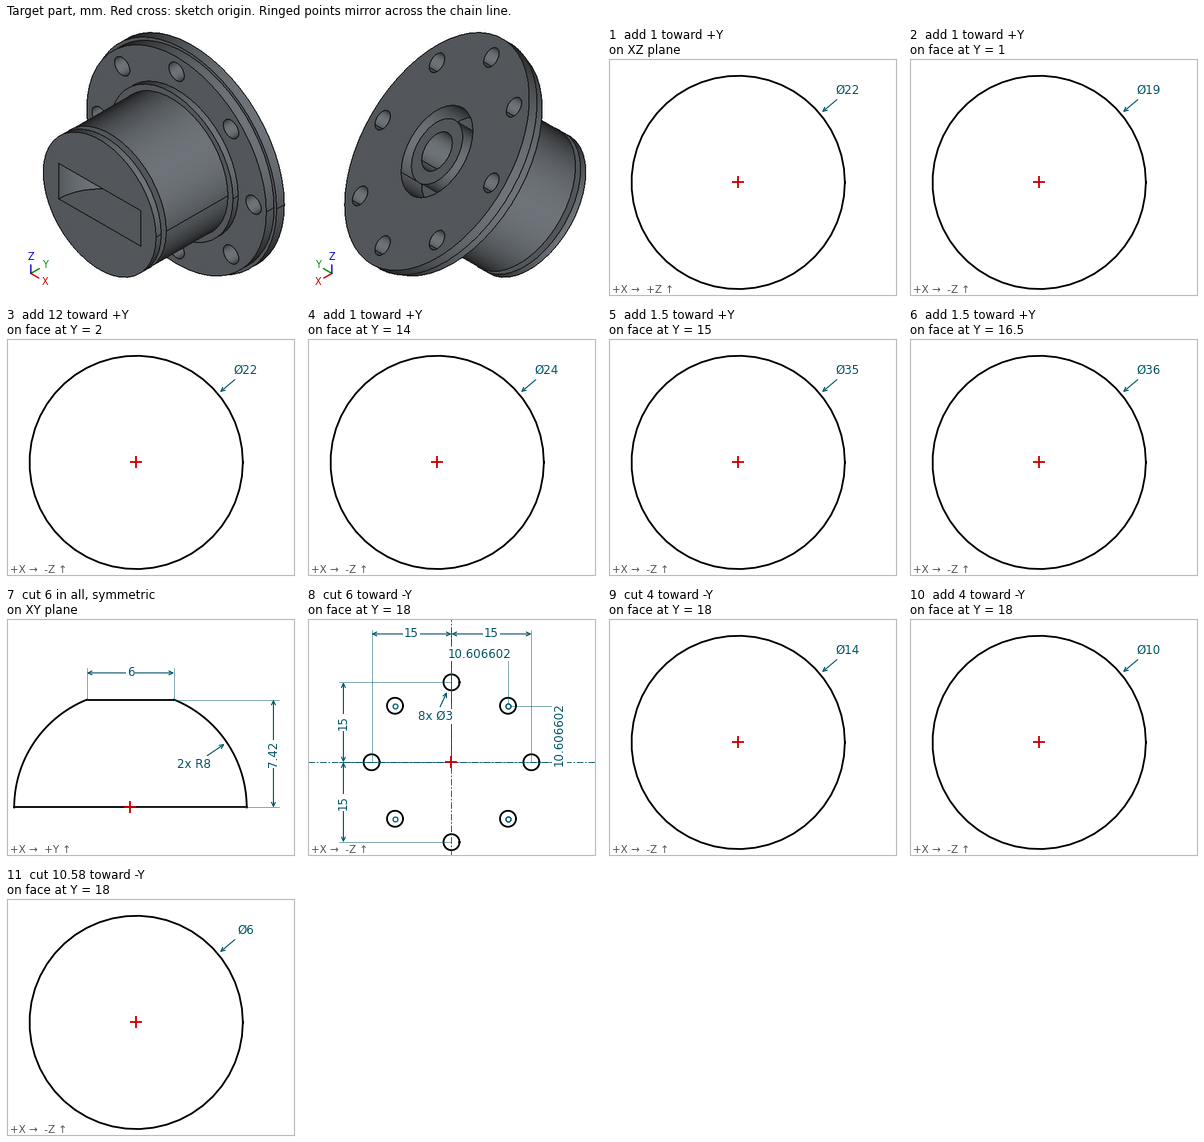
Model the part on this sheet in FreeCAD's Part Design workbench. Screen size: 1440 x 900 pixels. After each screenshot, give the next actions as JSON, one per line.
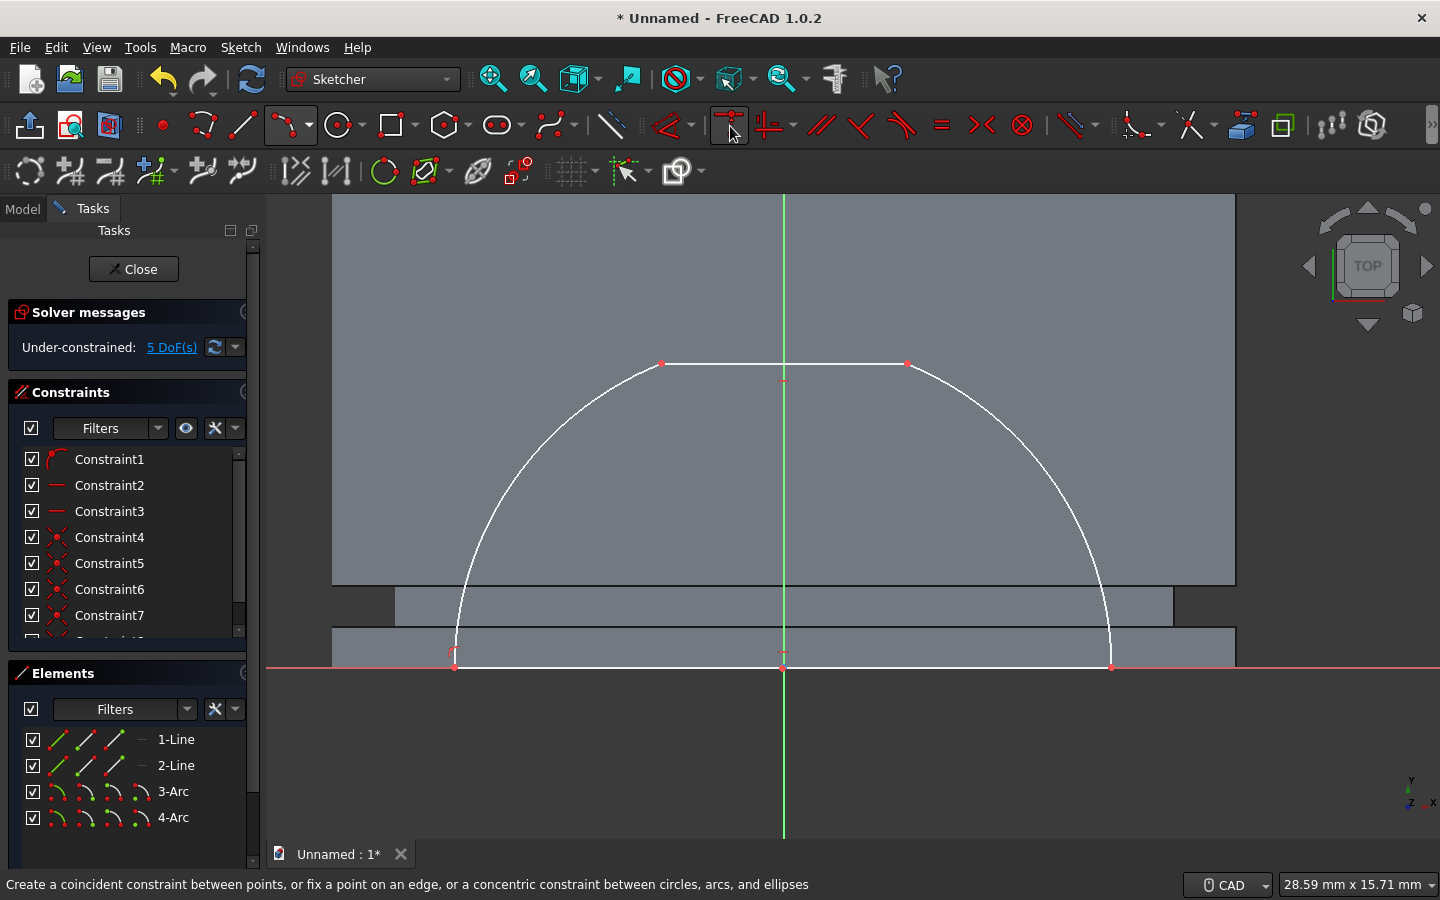
{"action": "left_click", "coordinate": [1091, 554]}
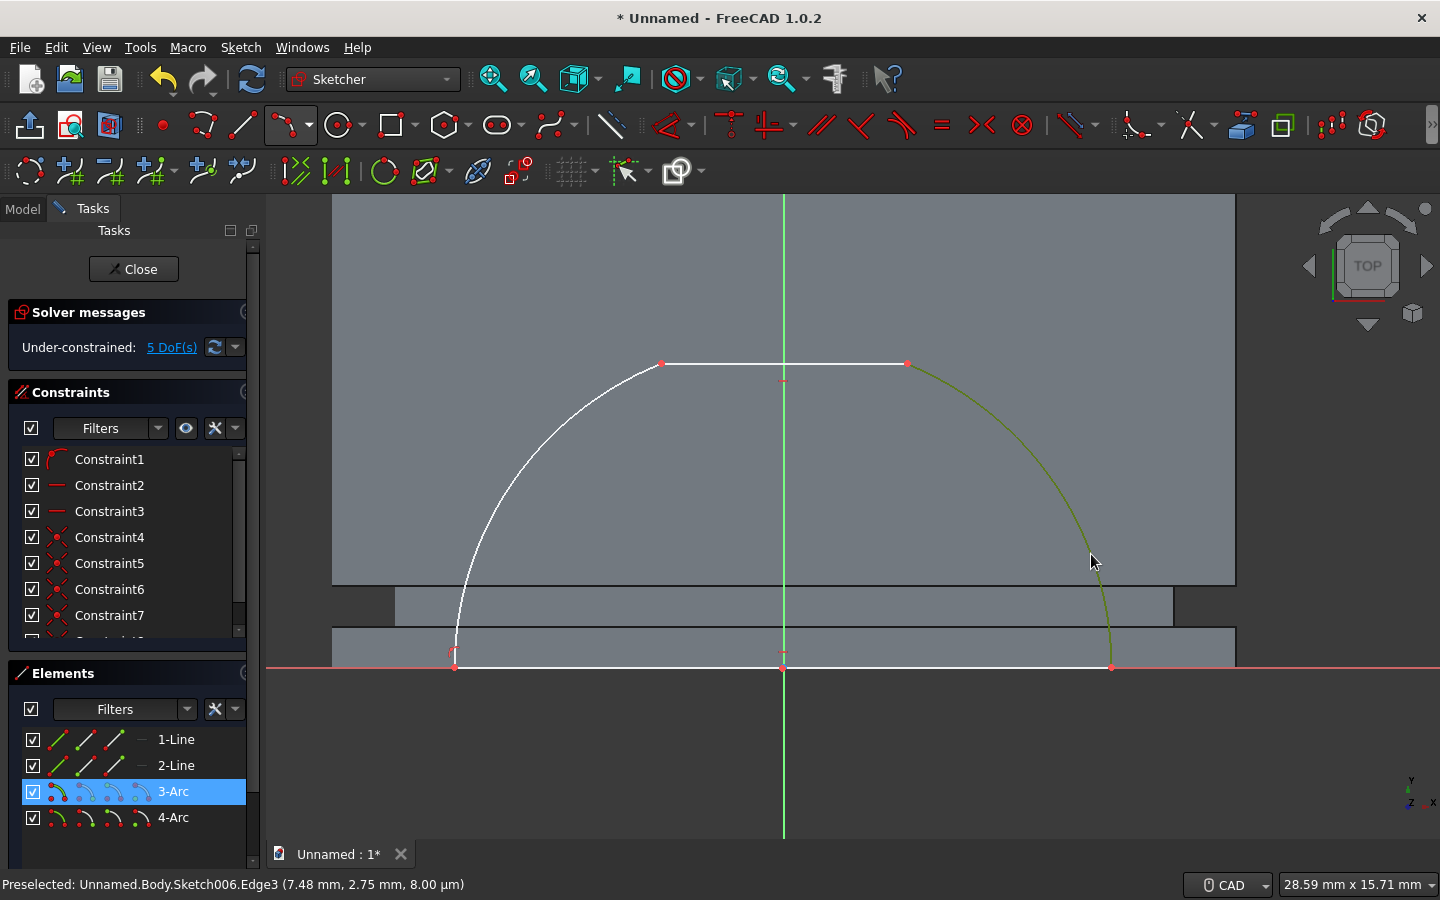
{"action": "left_click", "coordinate": [562, 426]}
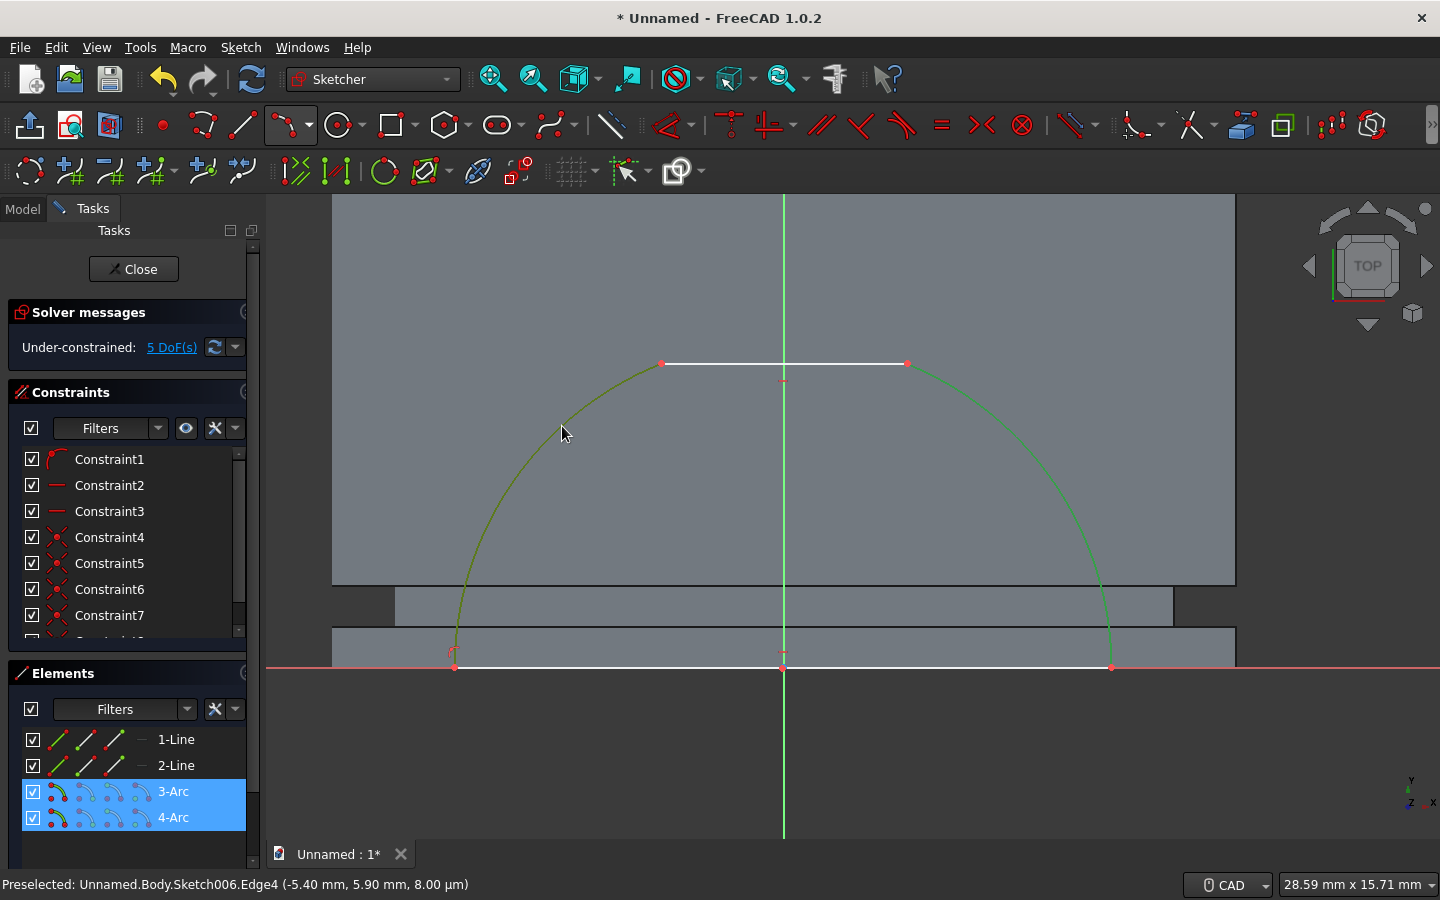
{"action": "left_click", "coordinate": [942, 126]}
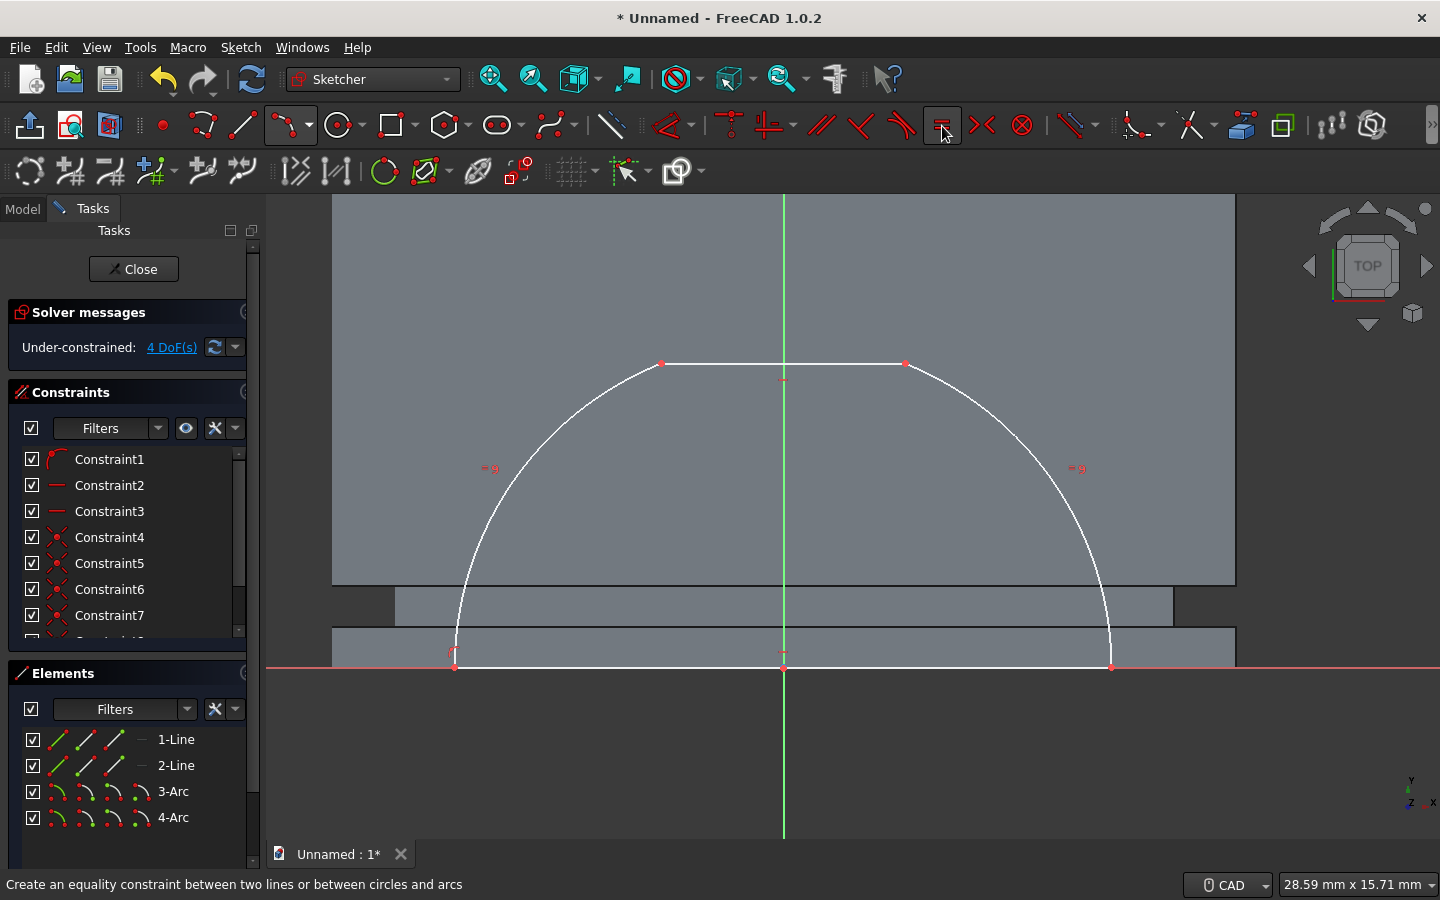
{"action": "scroll", "coordinate": [783, 669], "scroll_direction": "up", "scroll_amount": 13}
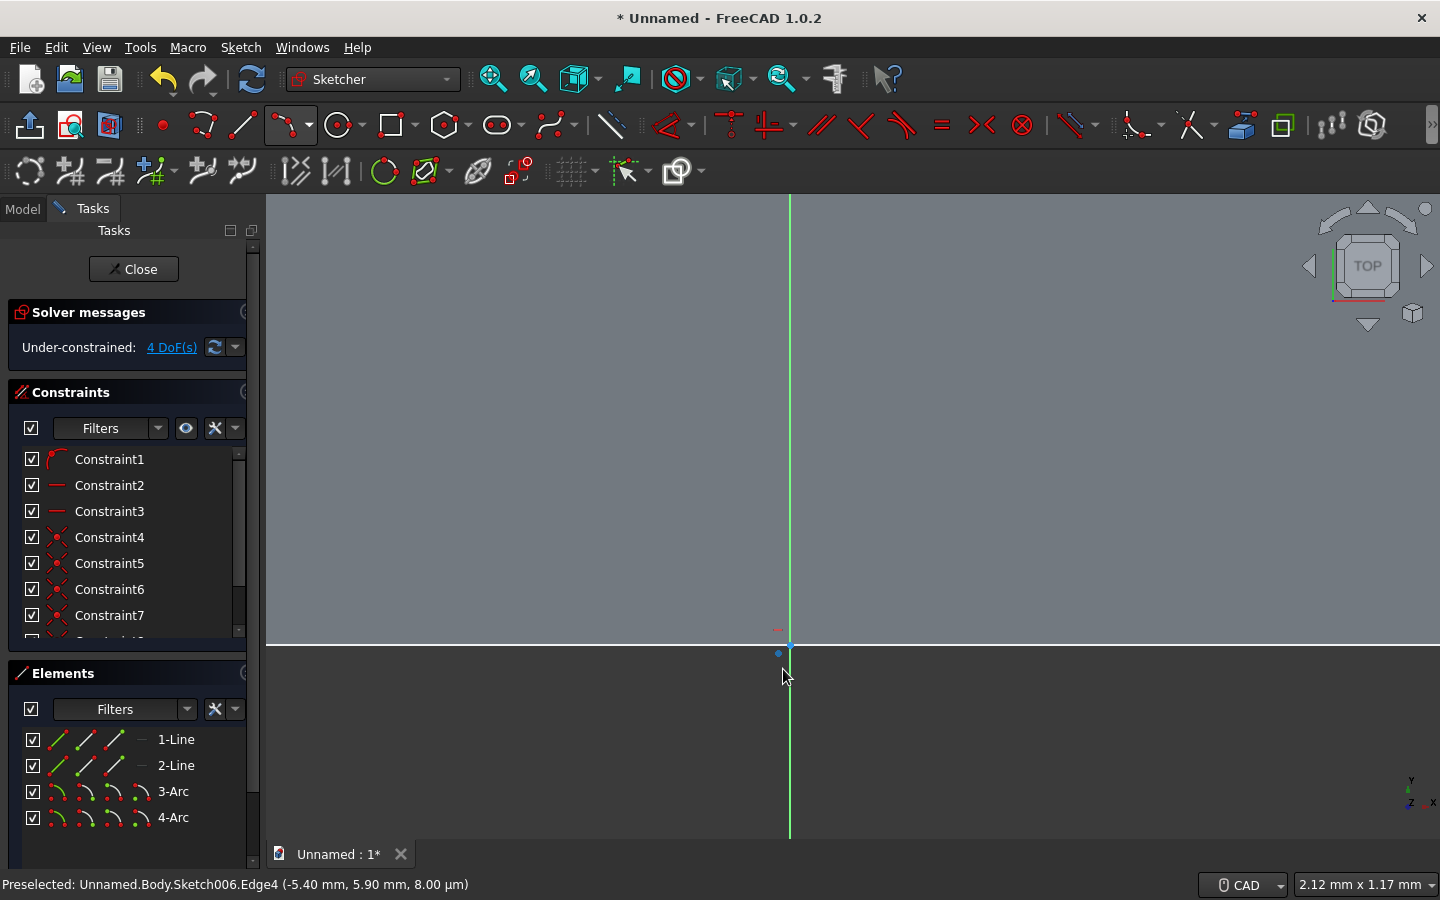
{"action": "left_click", "coordinate": [779, 653]}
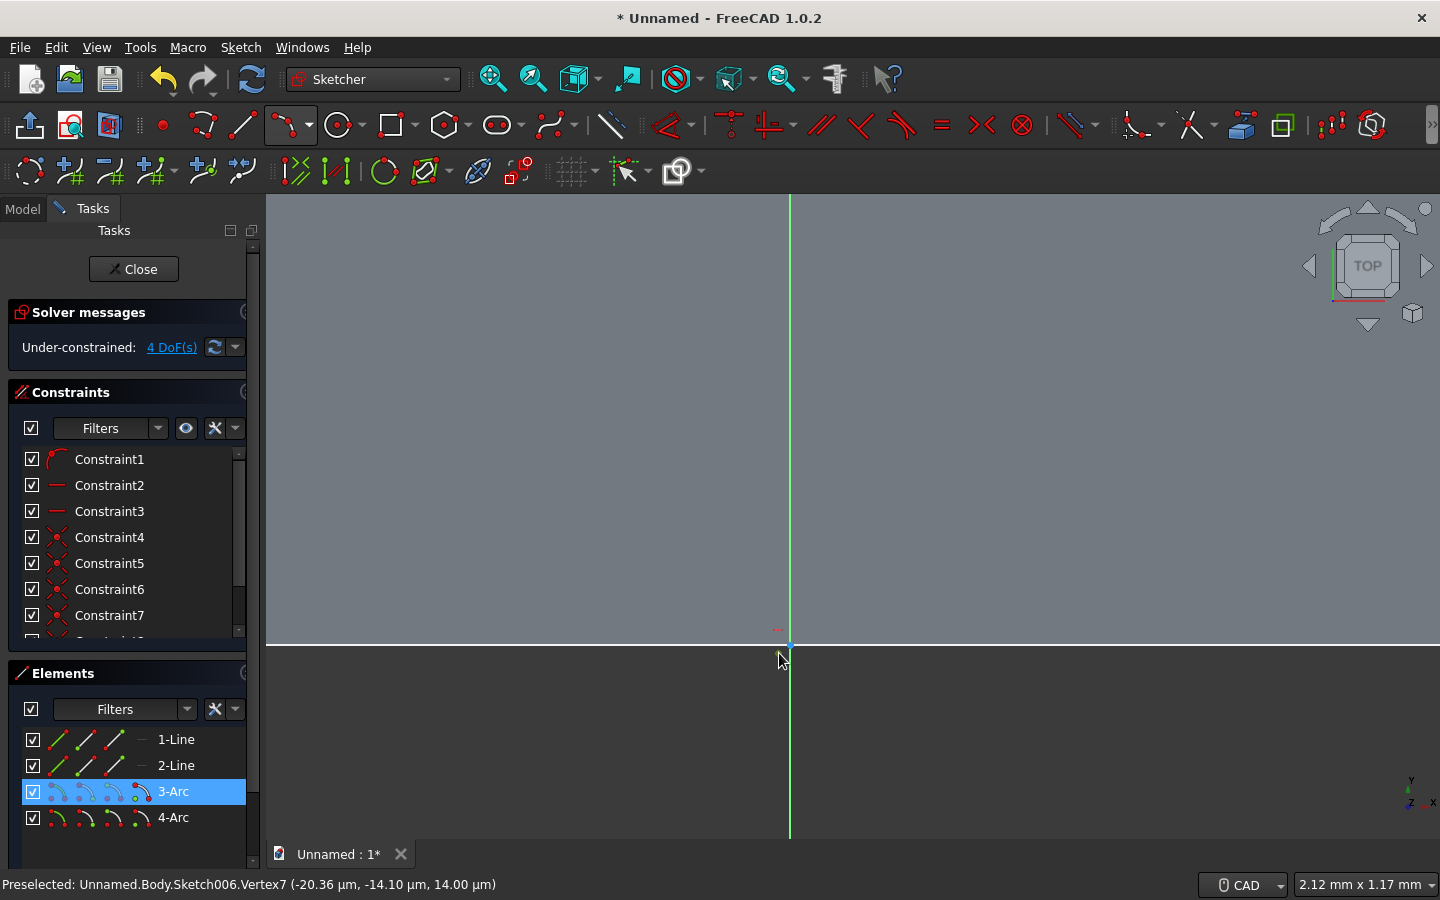
{"action": "left_click", "coordinate": [790, 769]}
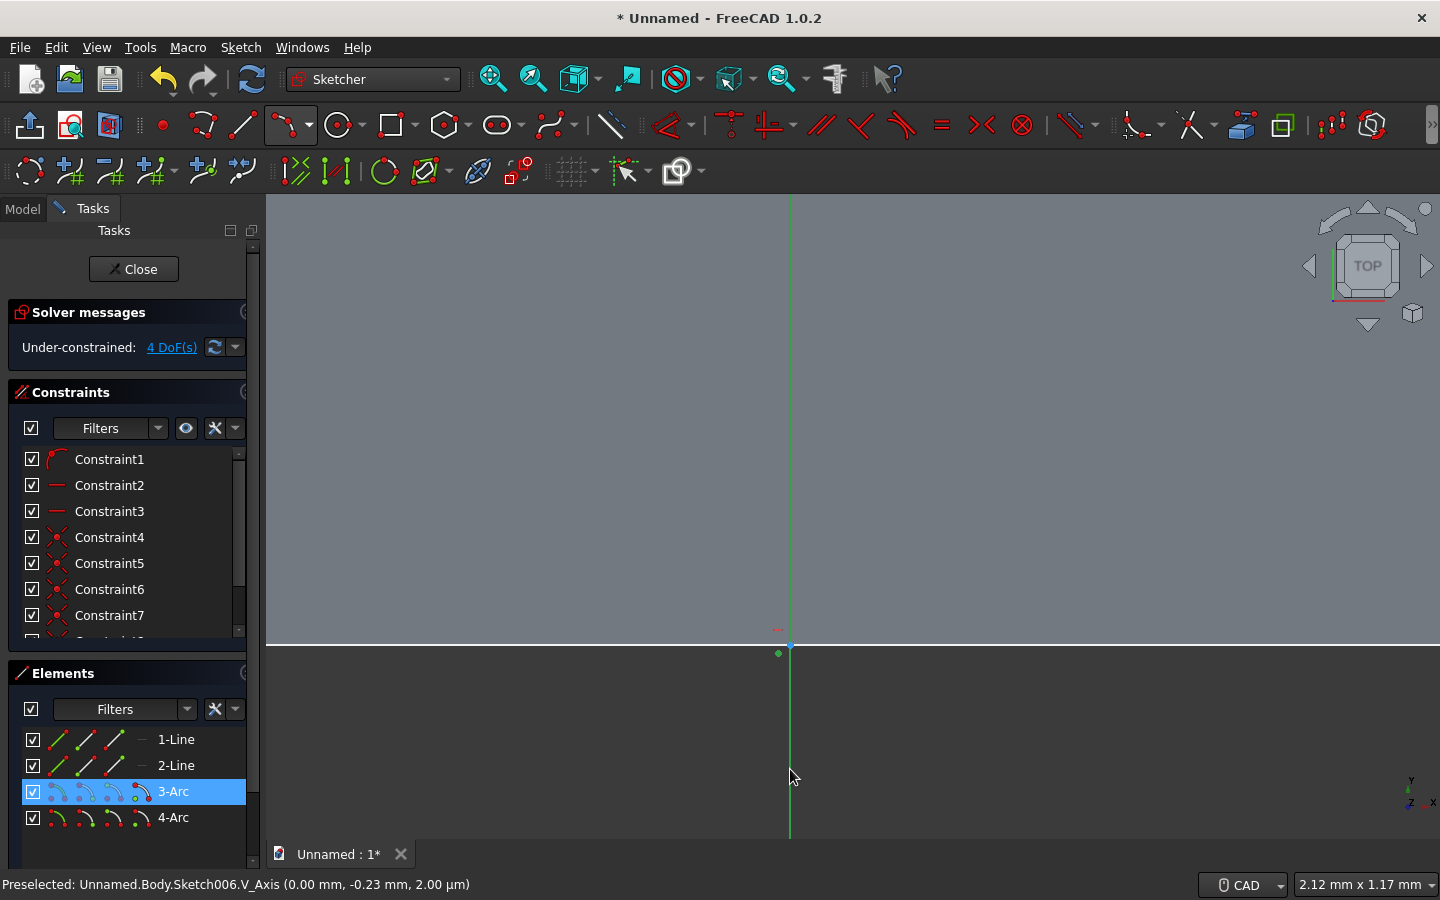
{"action": "left_click", "coordinate": [730, 126]}